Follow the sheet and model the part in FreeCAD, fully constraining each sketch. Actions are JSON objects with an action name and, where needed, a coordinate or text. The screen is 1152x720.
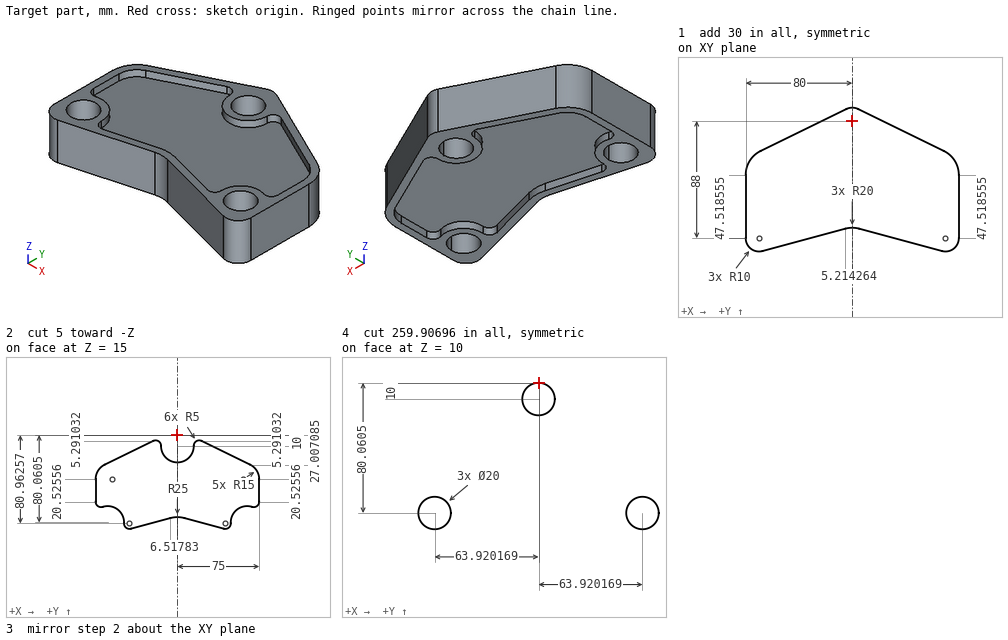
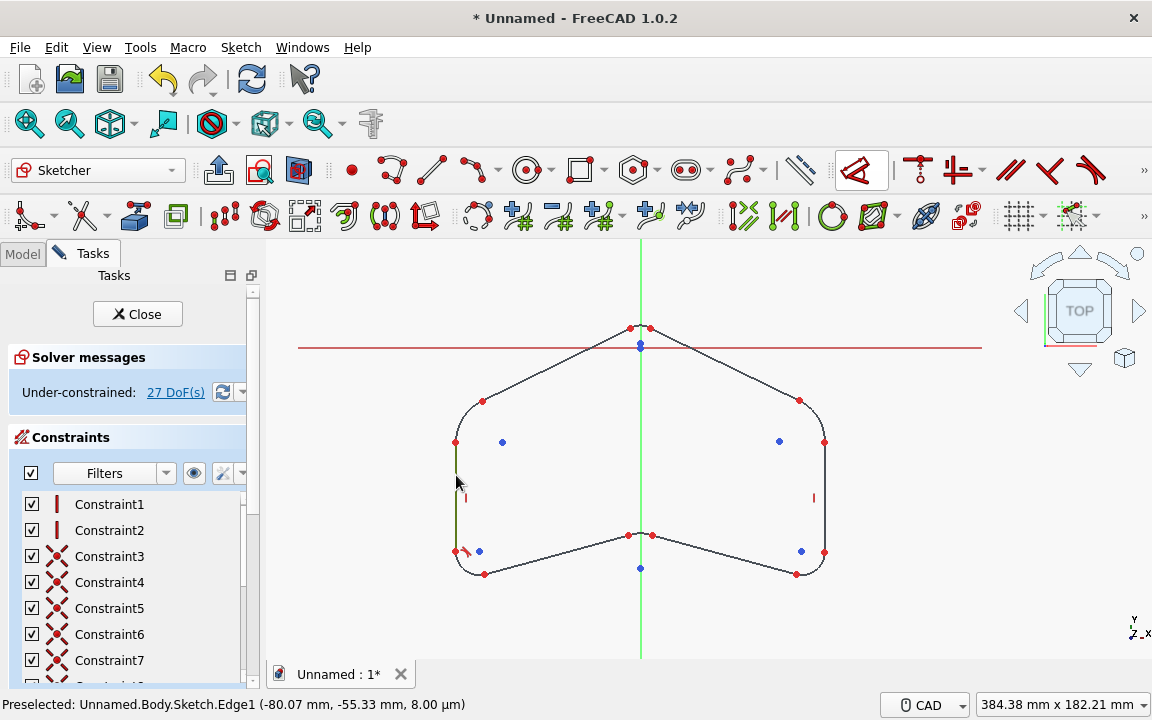
{"action": "left_click", "coordinate": [470, 410]}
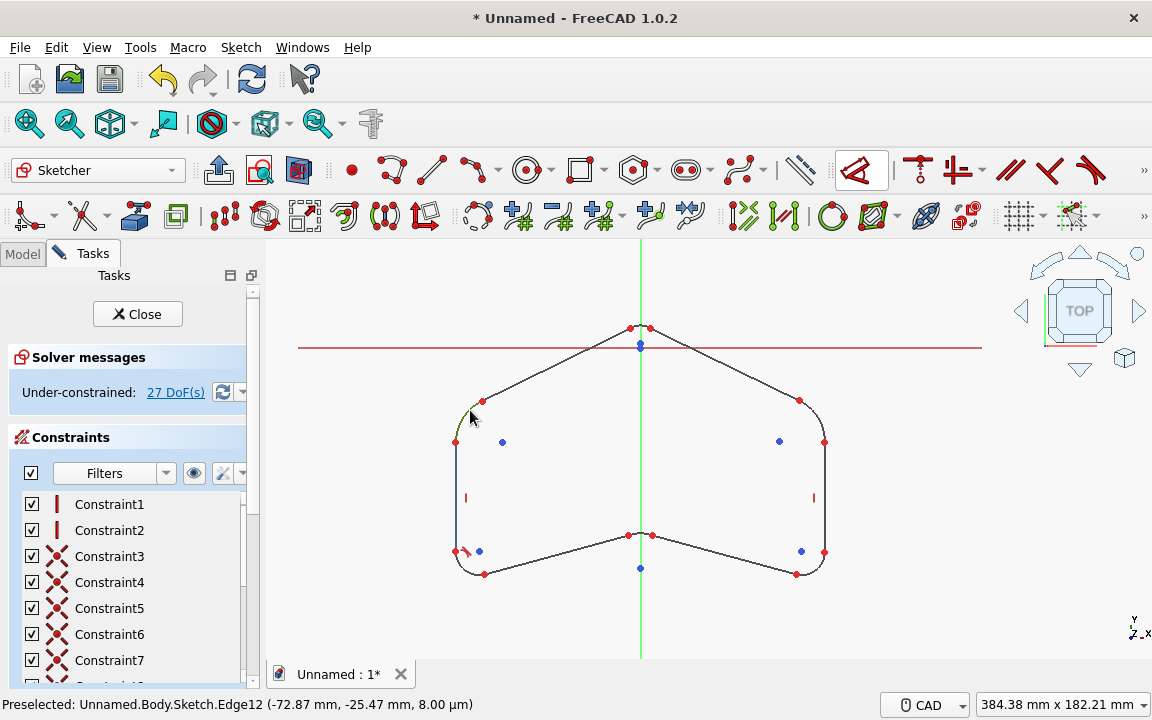
{"action": "key", "text": "t"}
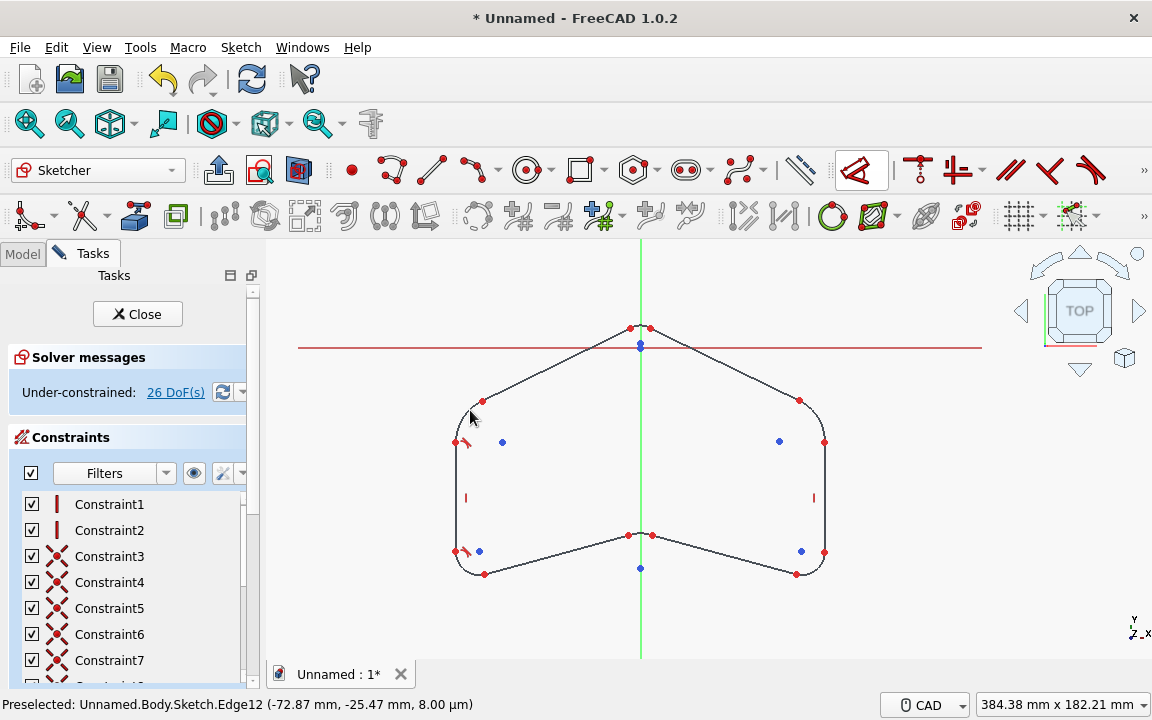
{"action": "left_click", "coordinate": [528, 563]}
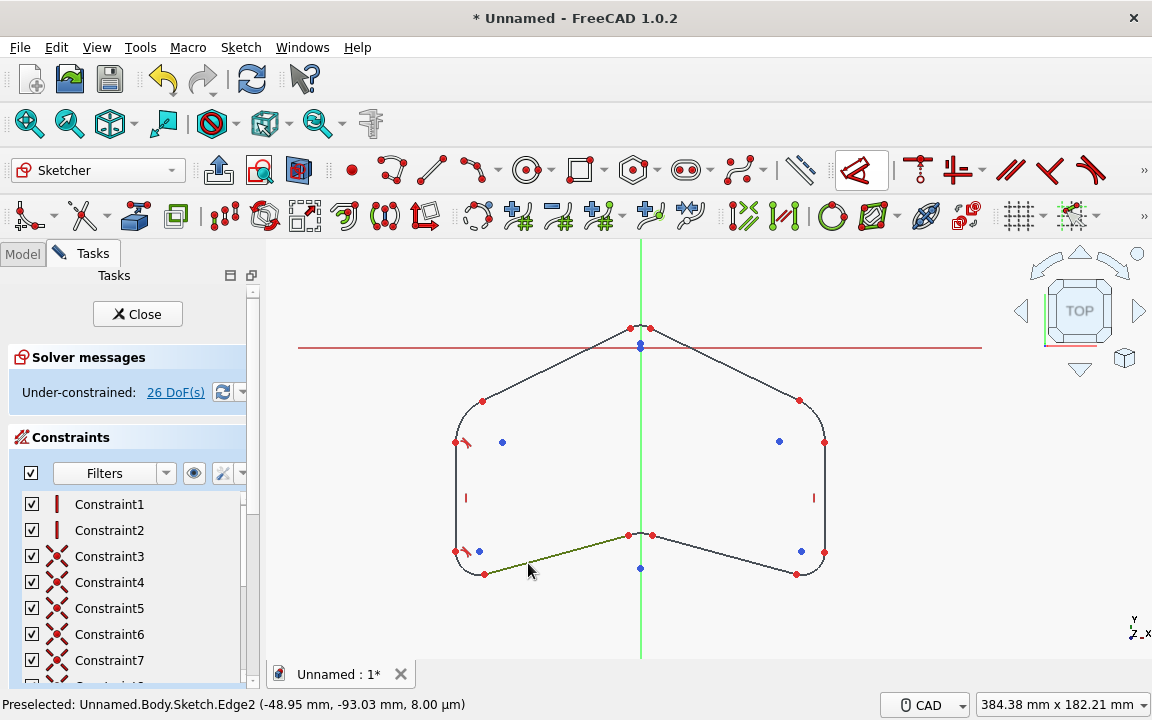
{"action": "left_click", "coordinate": [459, 564]}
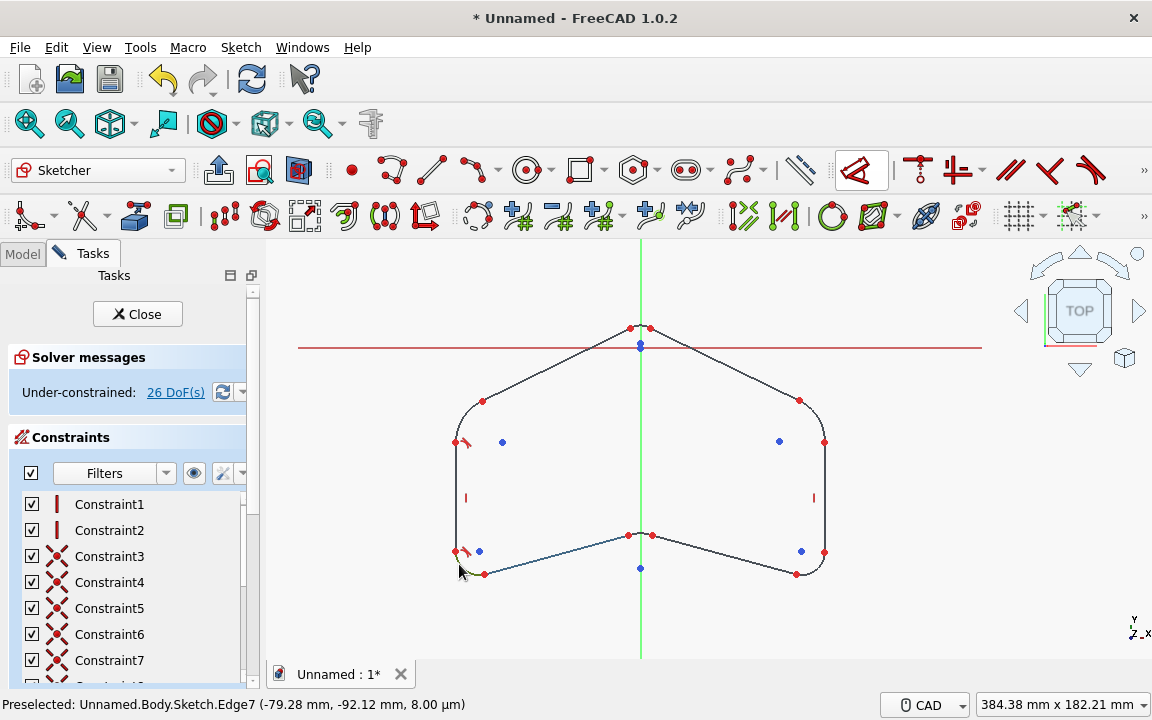
{"action": "left_click", "coordinate": [1092, 170]}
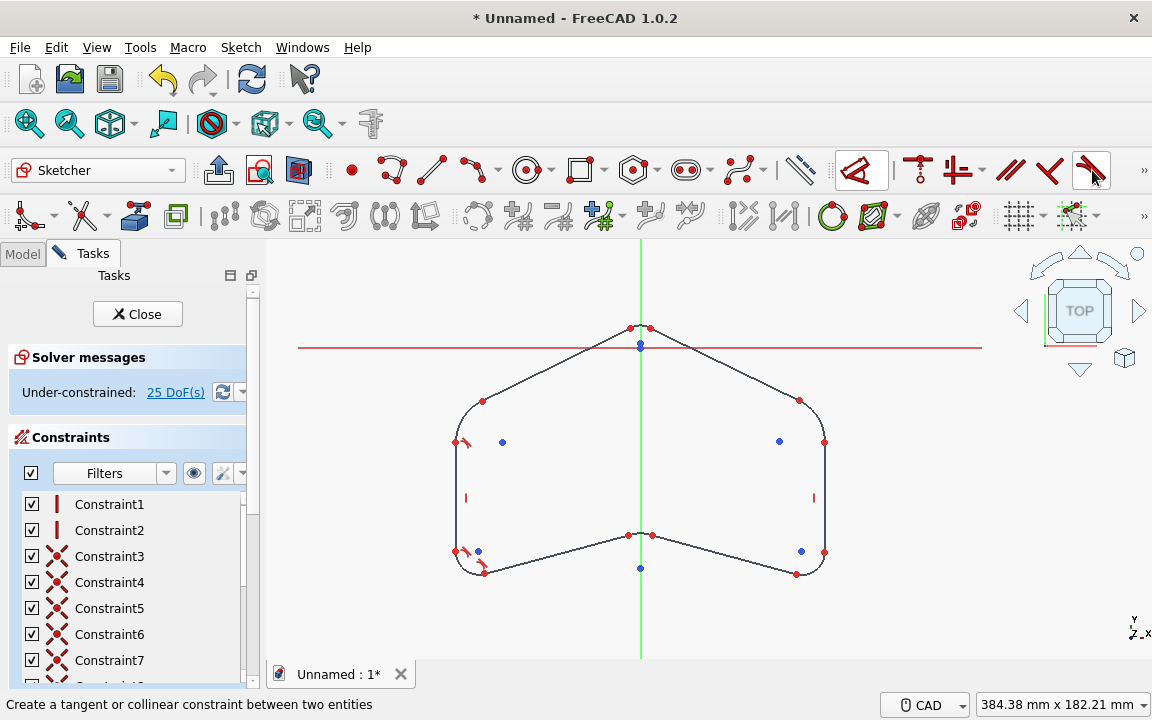
{"action": "left_click", "coordinate": [528, 562]}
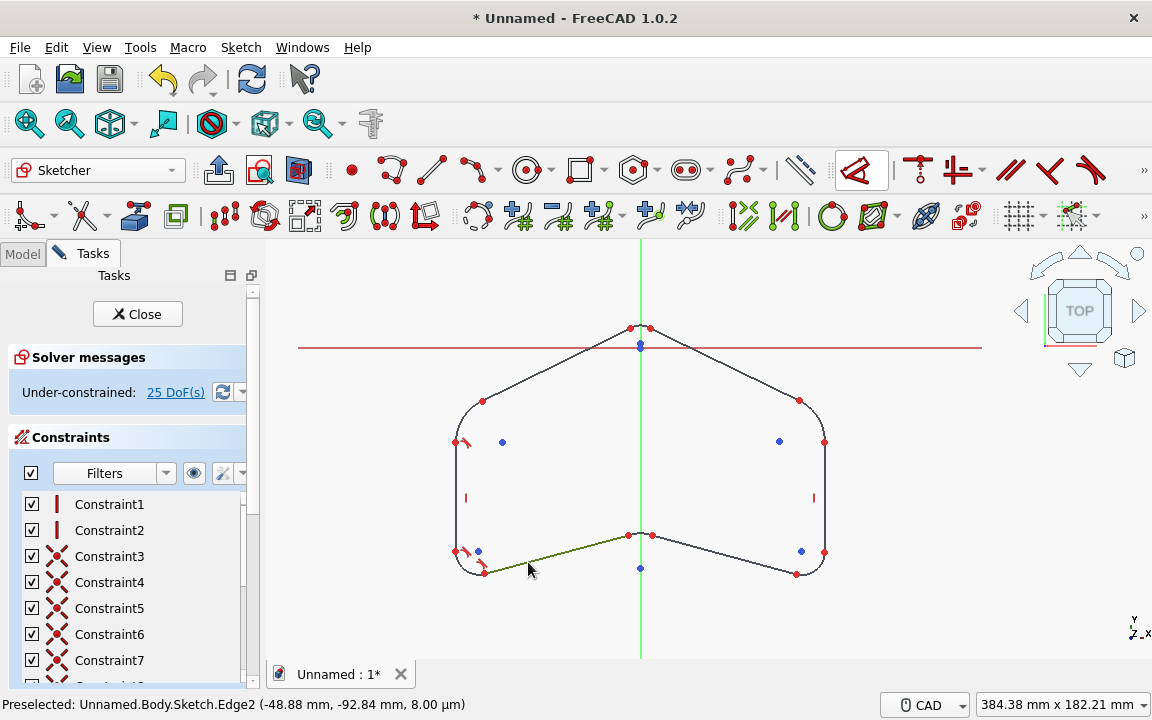
{"action": "left_click", "coordinate": [640, 533]}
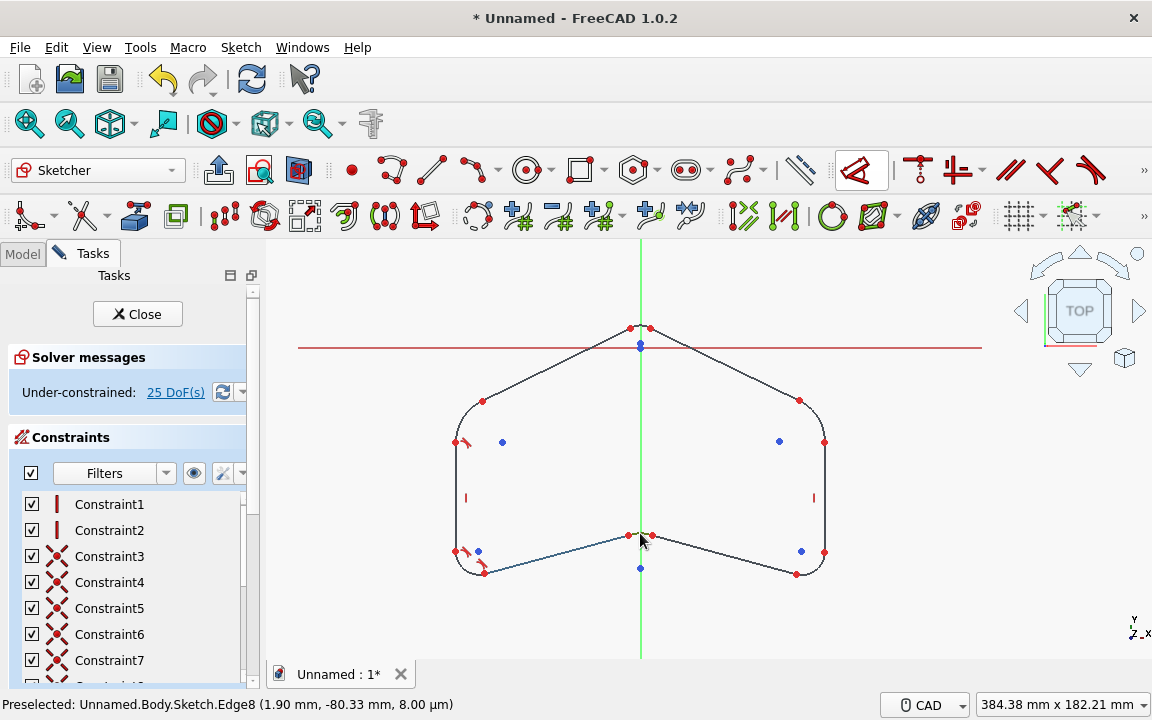
{"action": "left_click", "coordinate": [1092, 170]}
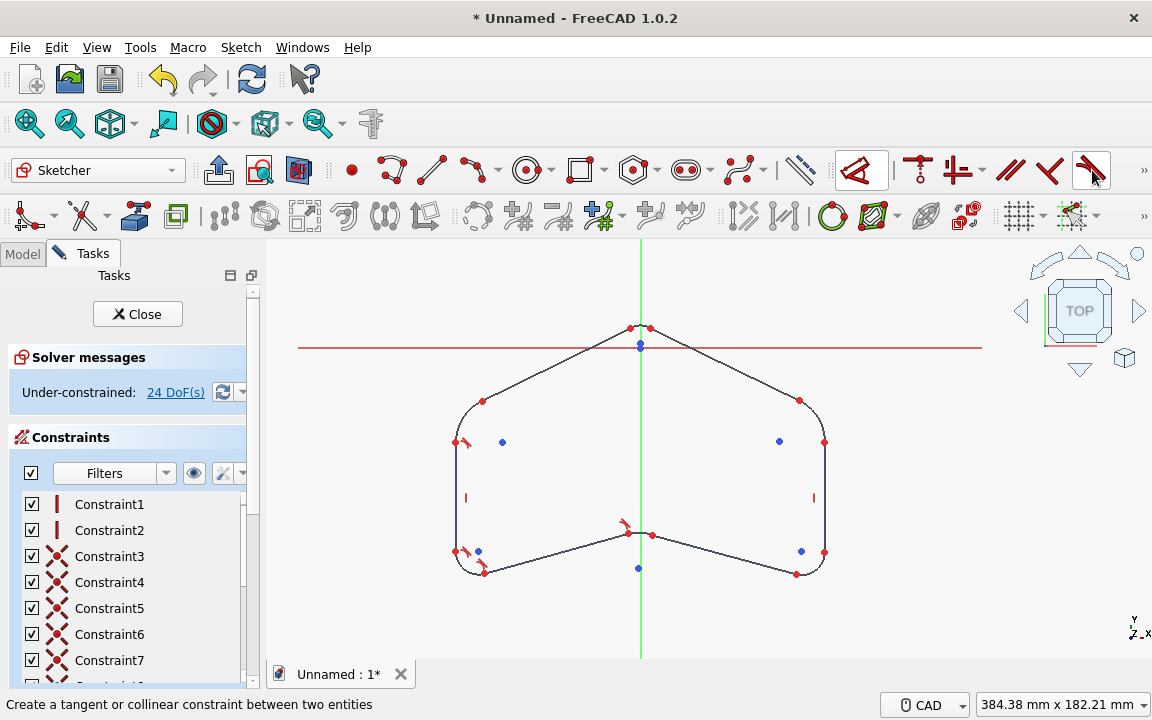
{"action": "left_click", "coordinate": [696, 547]}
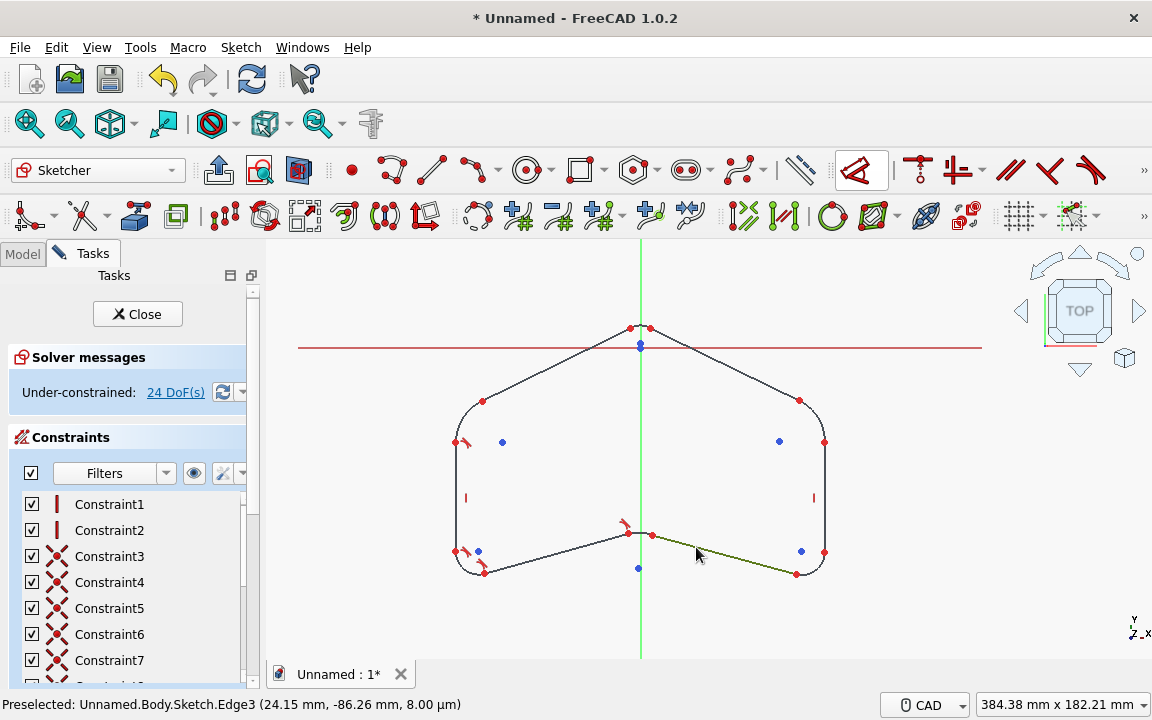
{"action": "left_click", "coordinate": [641, 533]}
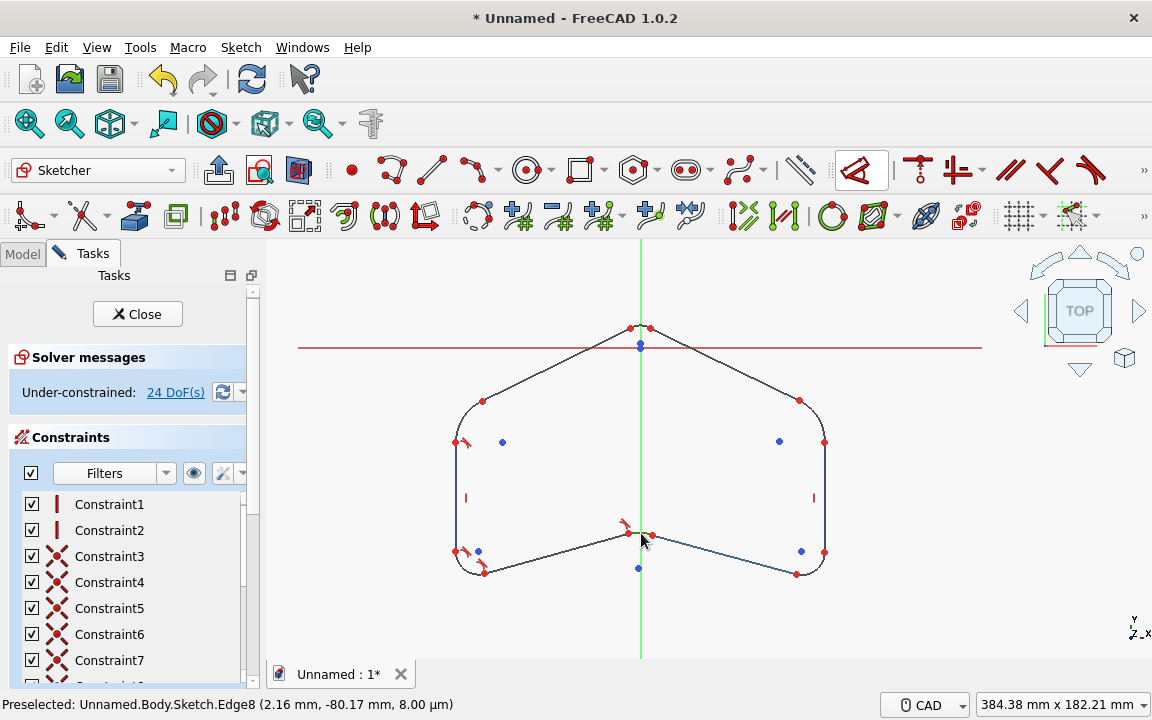
{"action": "left_click", "coordinate": [1092, 170]}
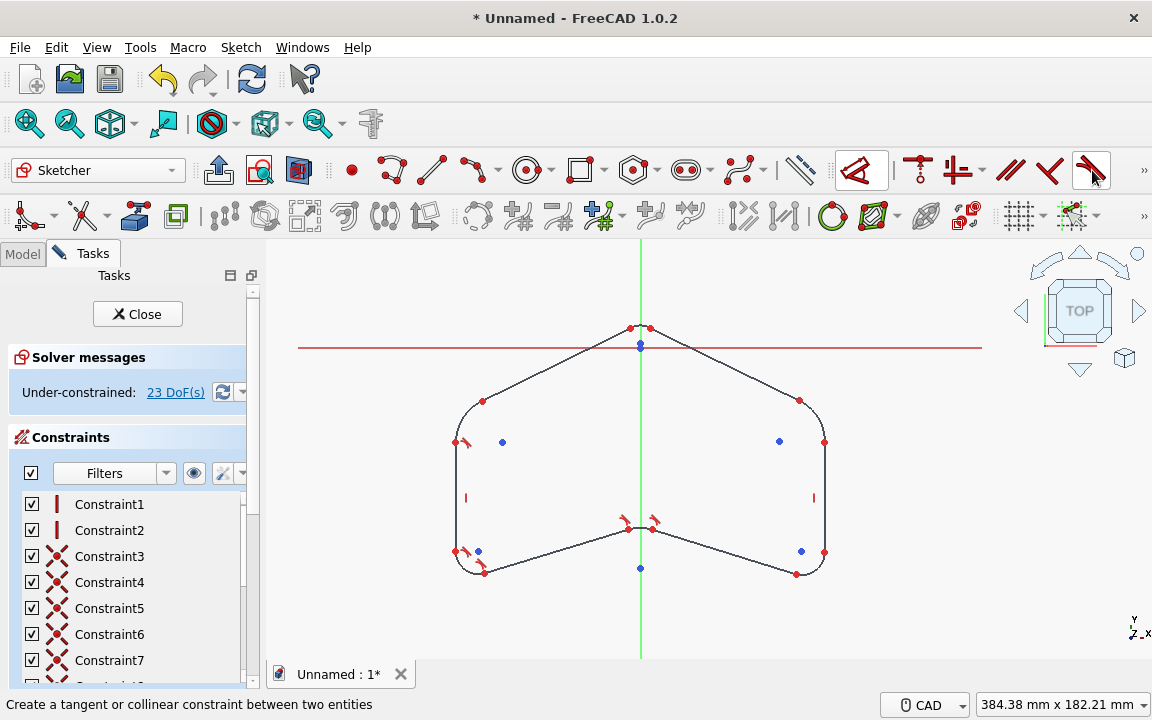
{"action": "left_click", "coordinate": [696, 543]}